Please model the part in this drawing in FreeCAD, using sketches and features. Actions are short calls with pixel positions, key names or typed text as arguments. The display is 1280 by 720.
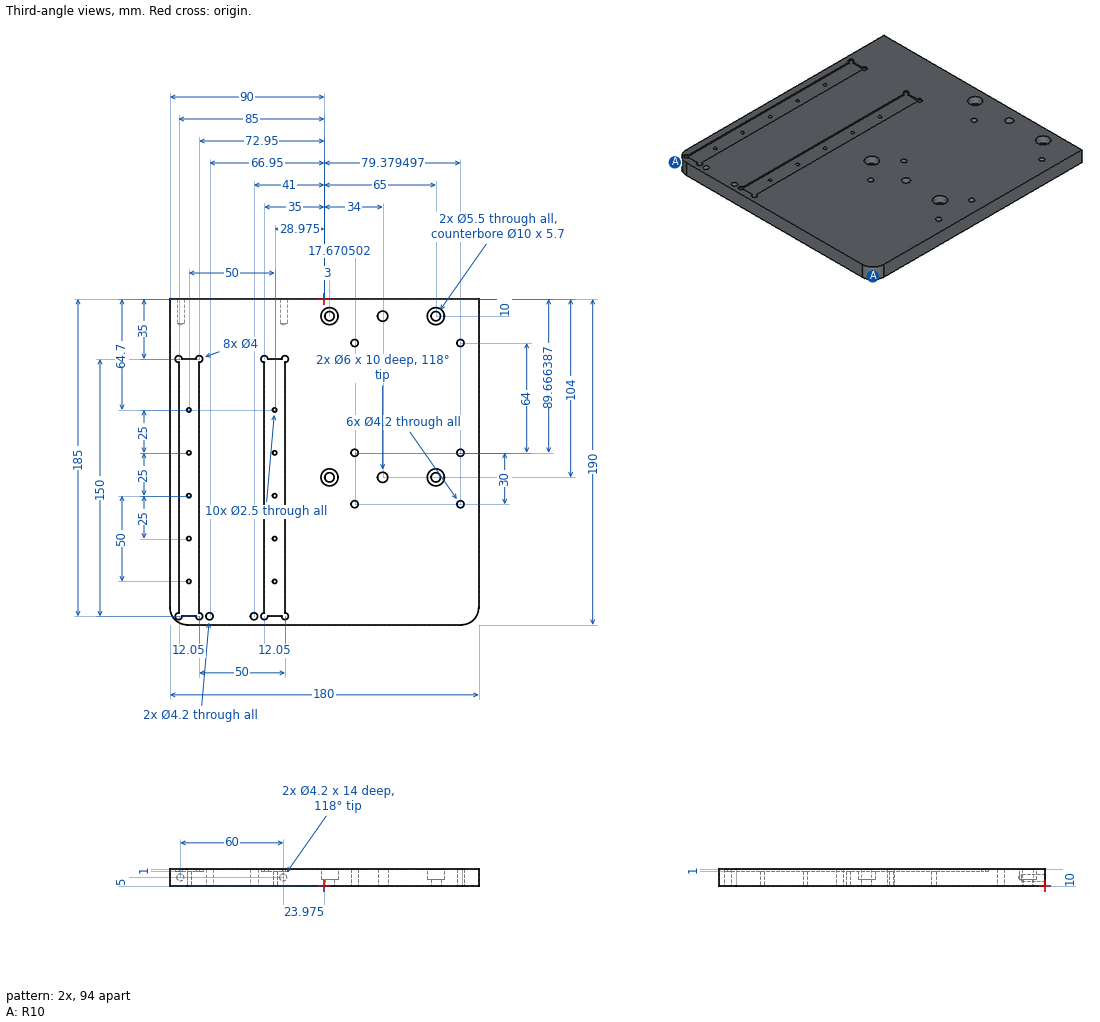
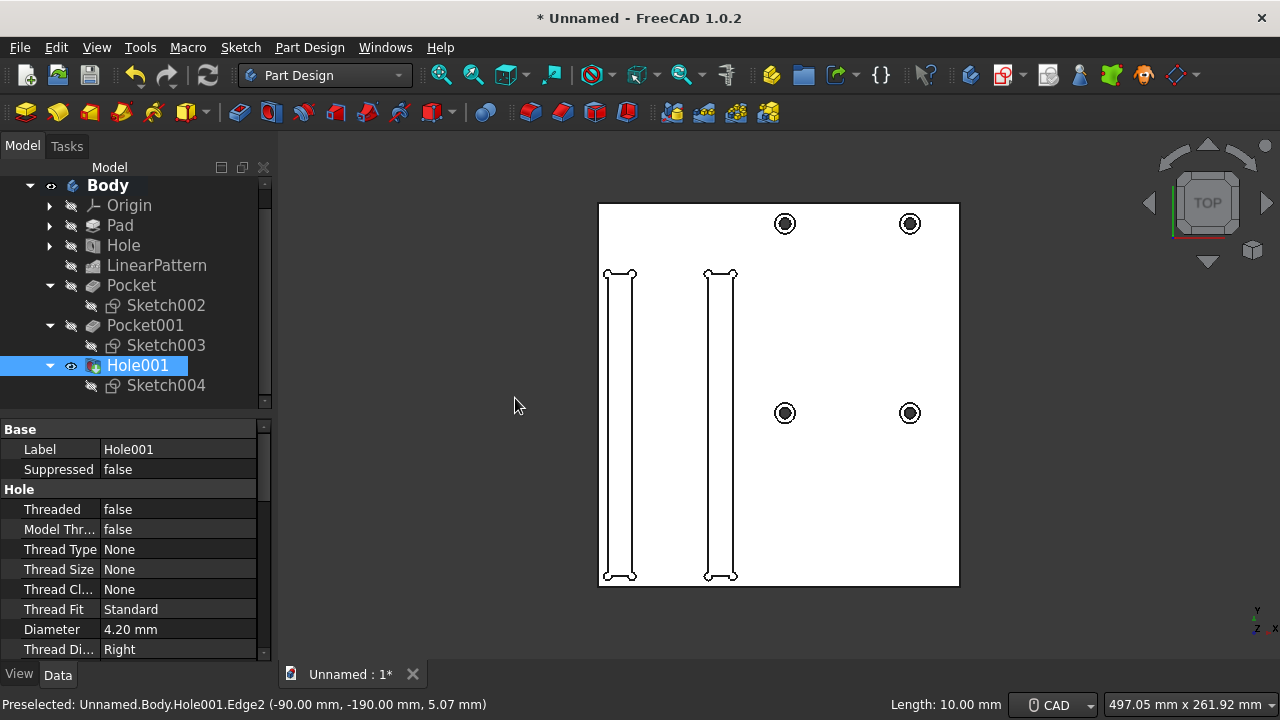
scroll(598, 586, up, 4)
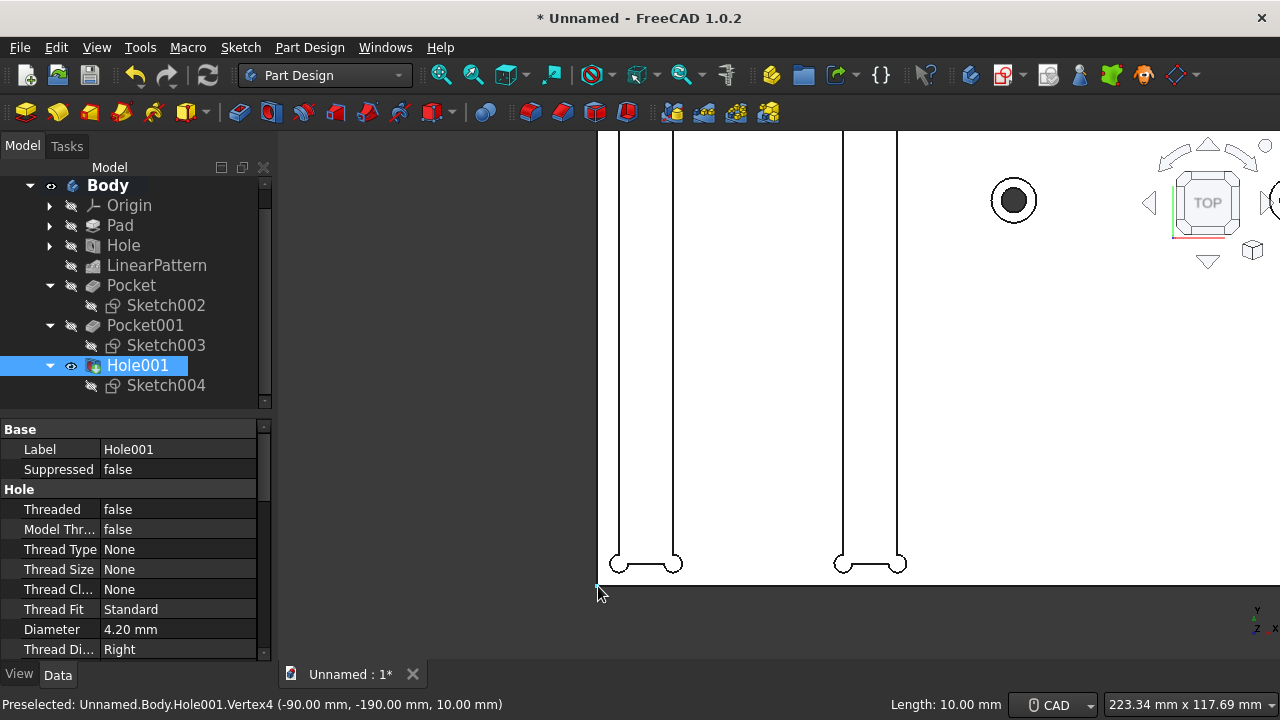
click(442, 76)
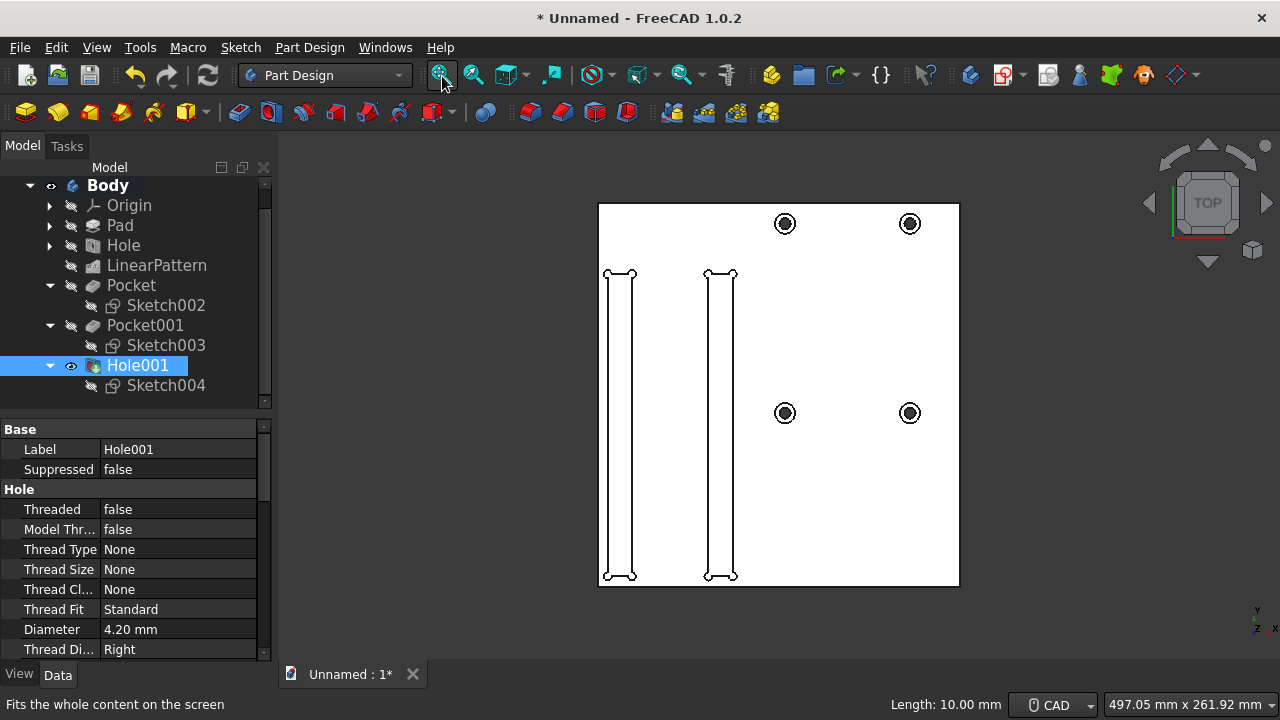
key(1)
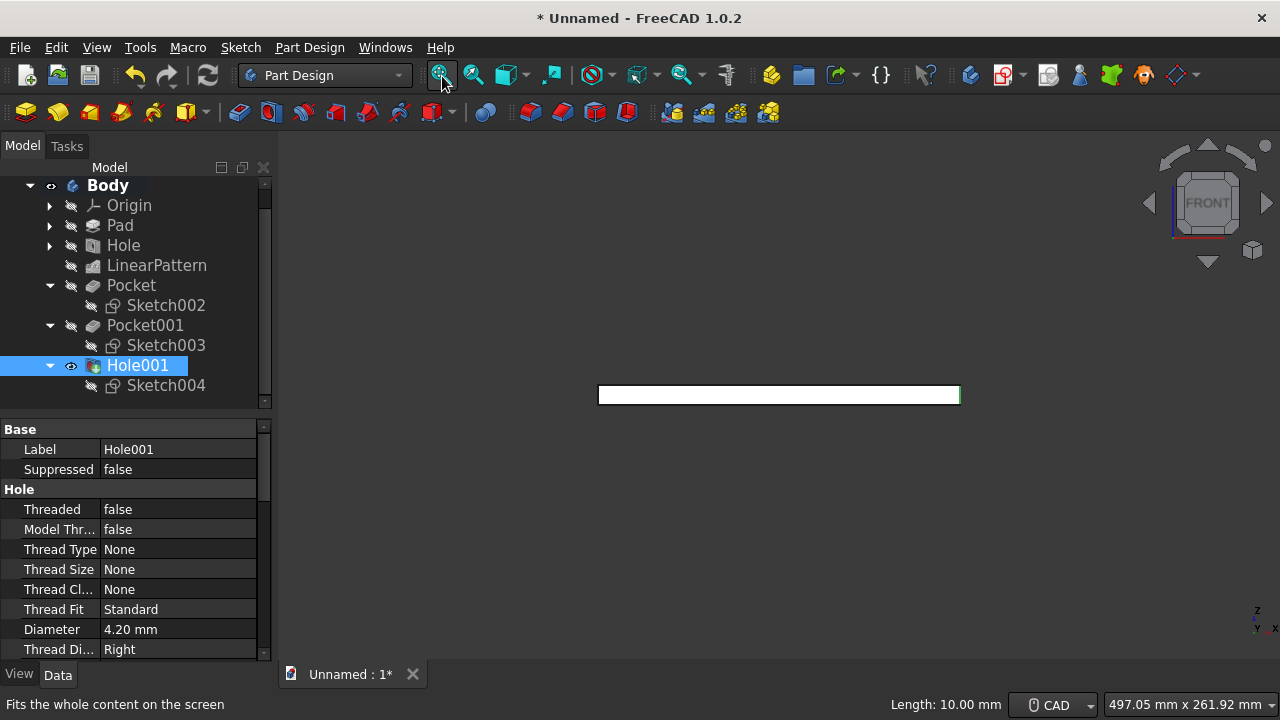
click(442, 76)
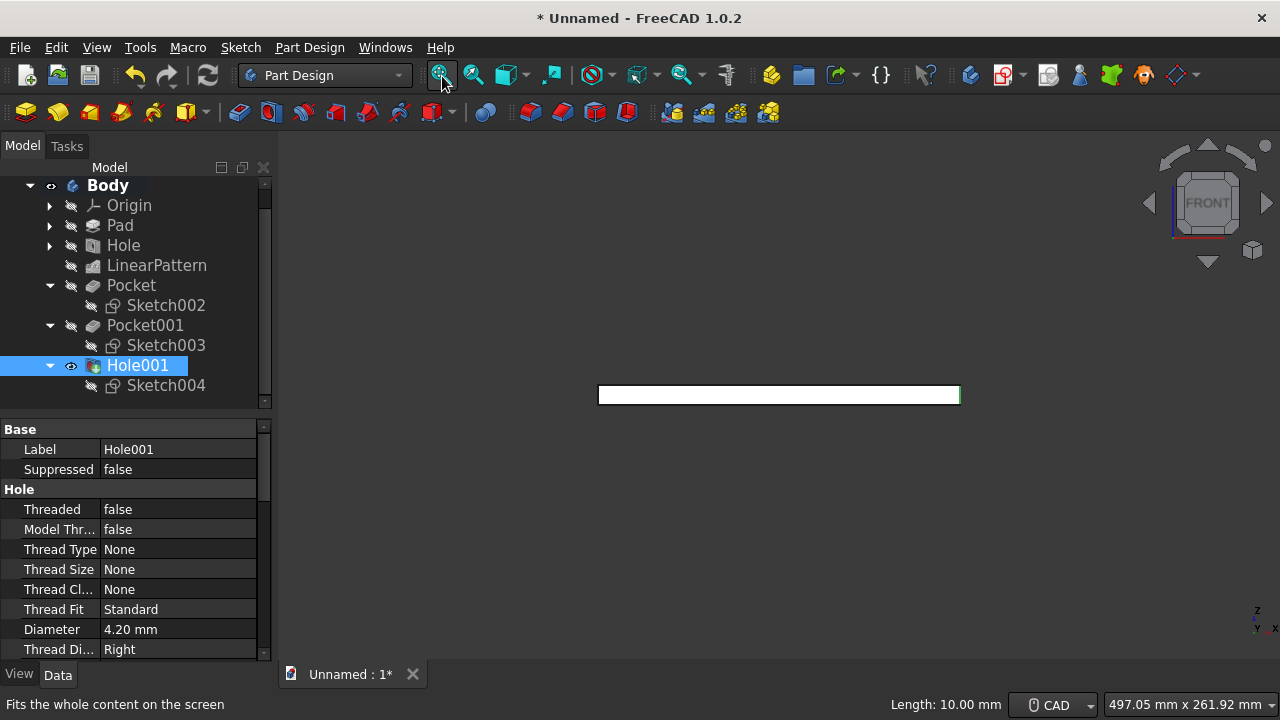
click(598, 394, ctrl)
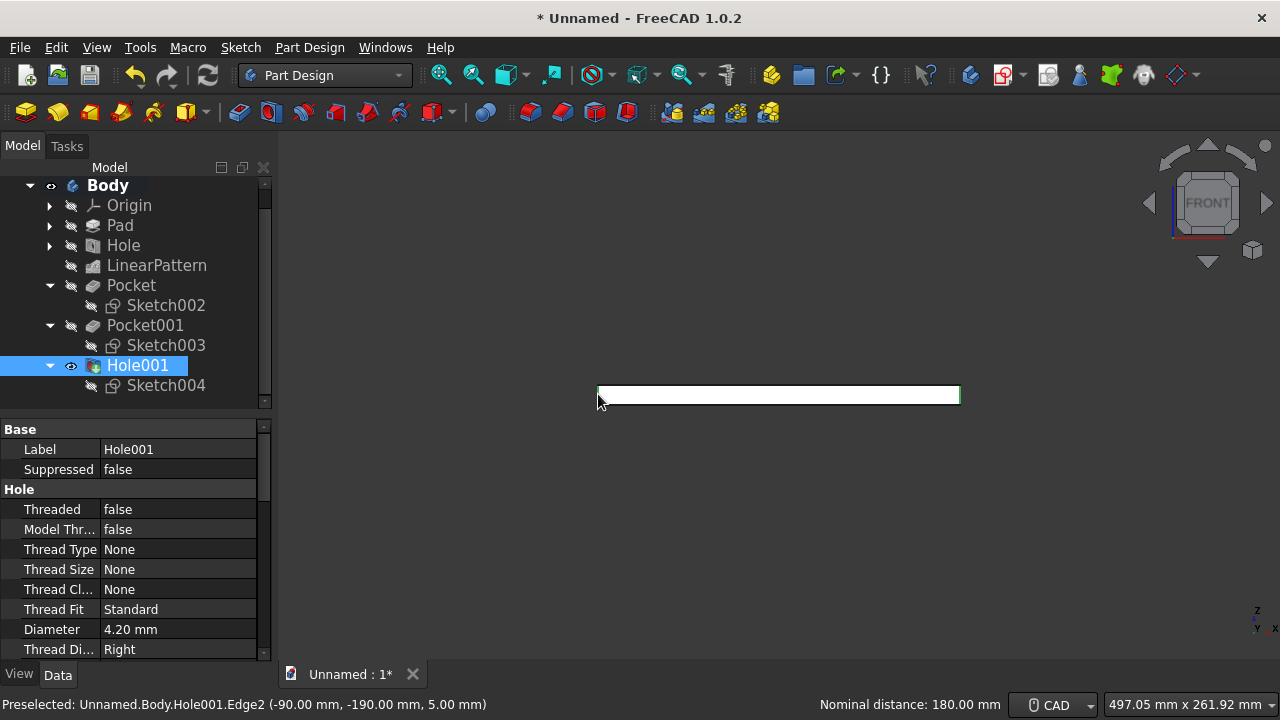
click(532, 112)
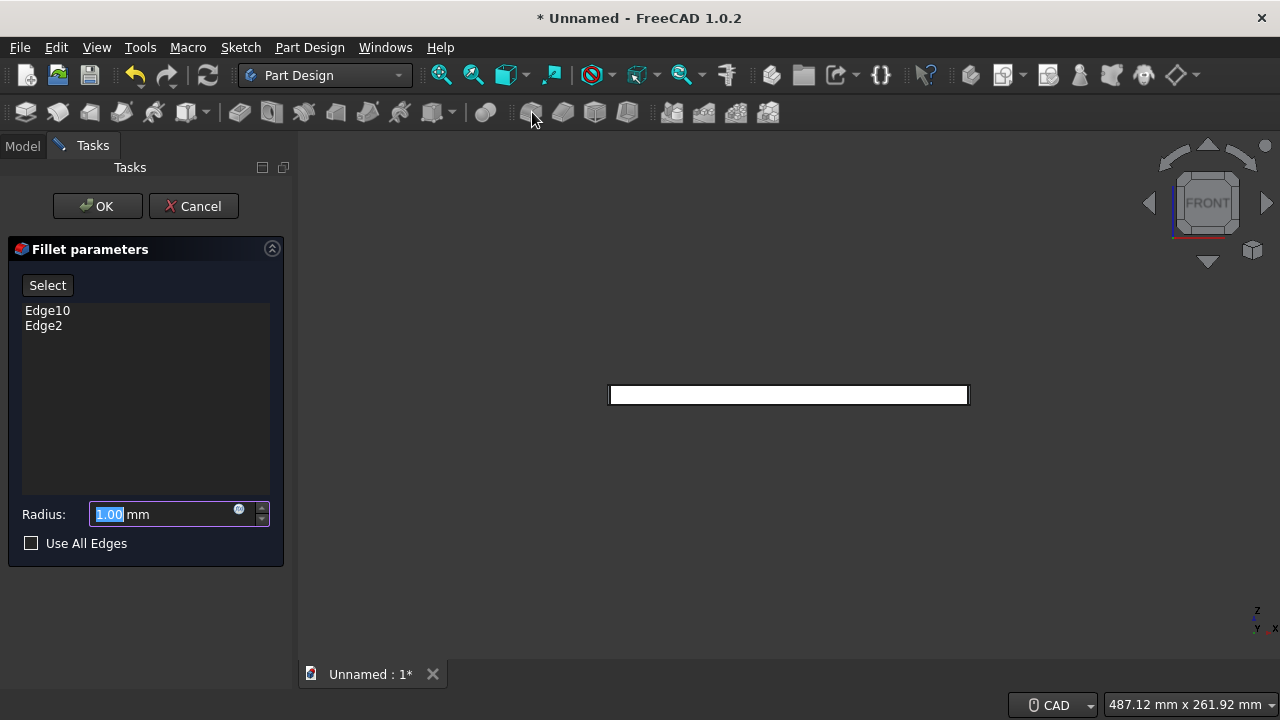
text(10)
key(Tab)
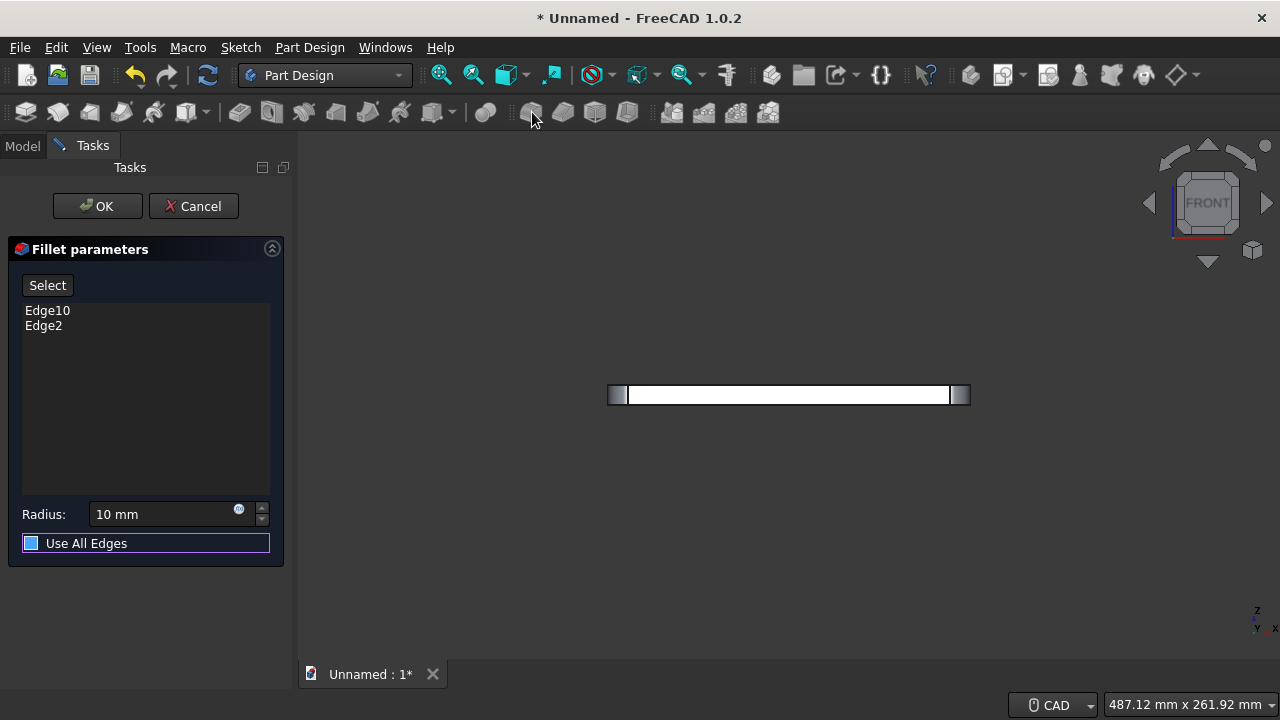
click(98, 206)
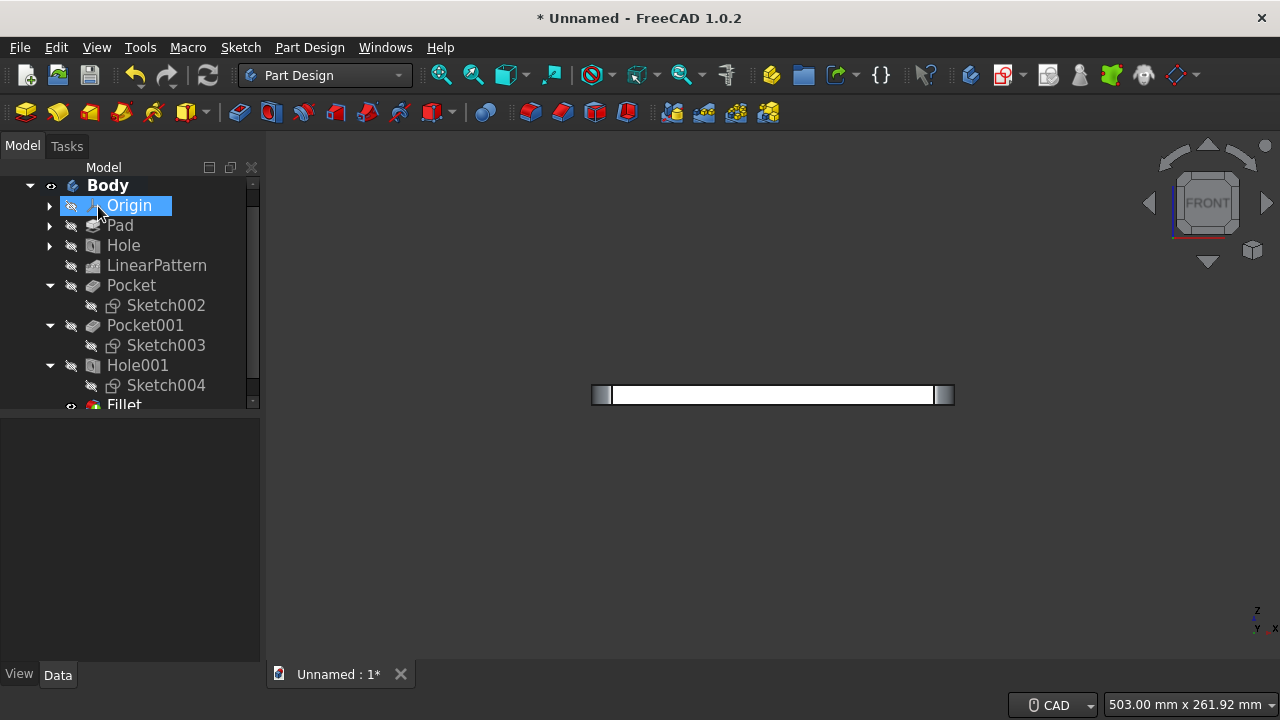
key(v)
key(f)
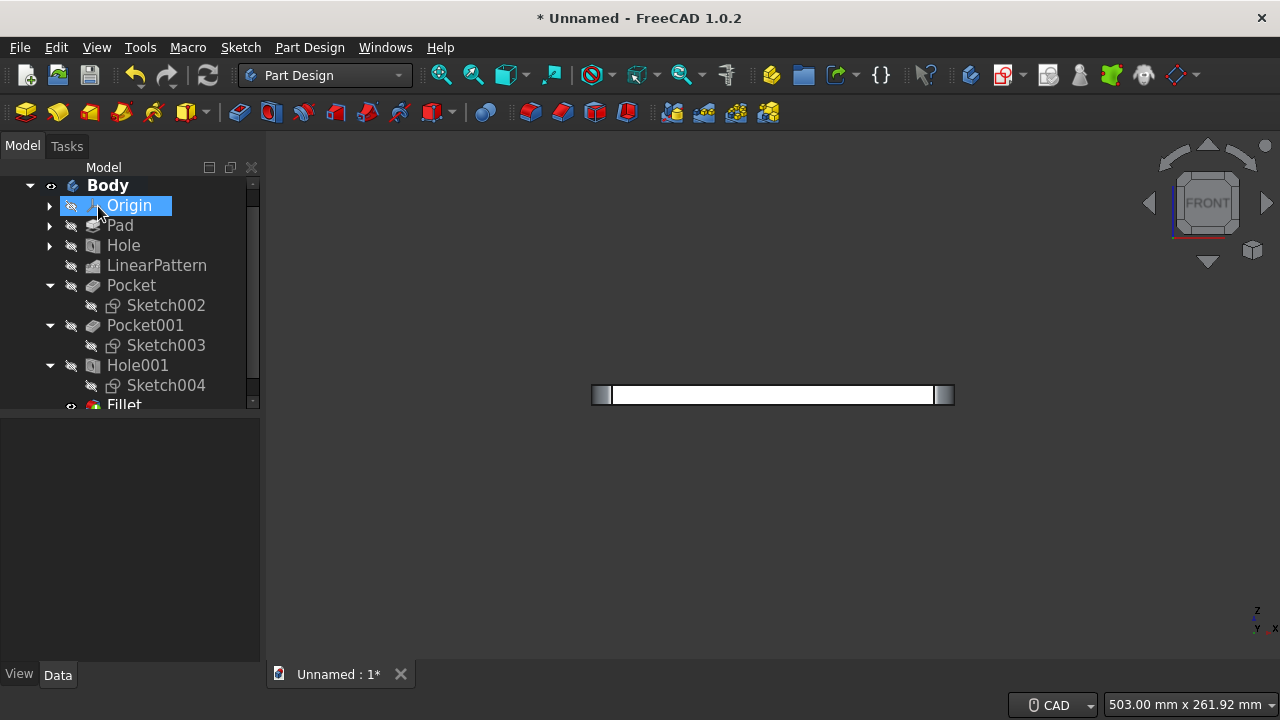
key(0)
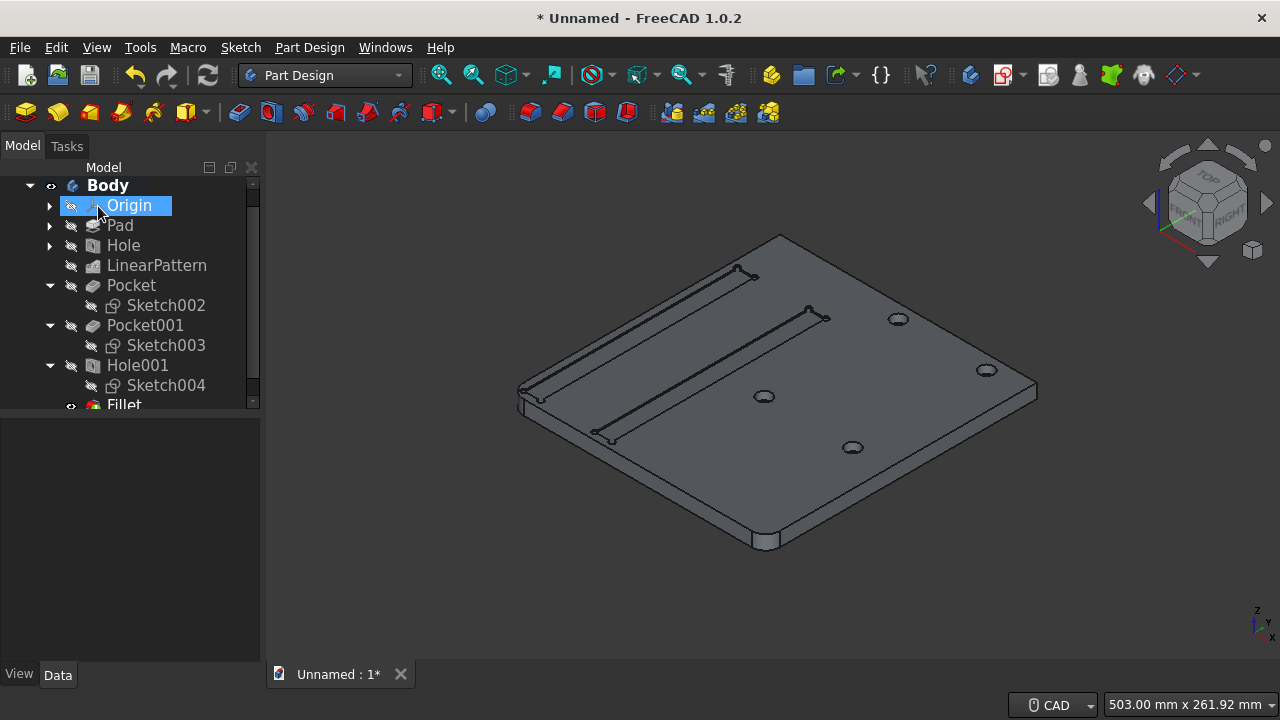
click(732, 452)